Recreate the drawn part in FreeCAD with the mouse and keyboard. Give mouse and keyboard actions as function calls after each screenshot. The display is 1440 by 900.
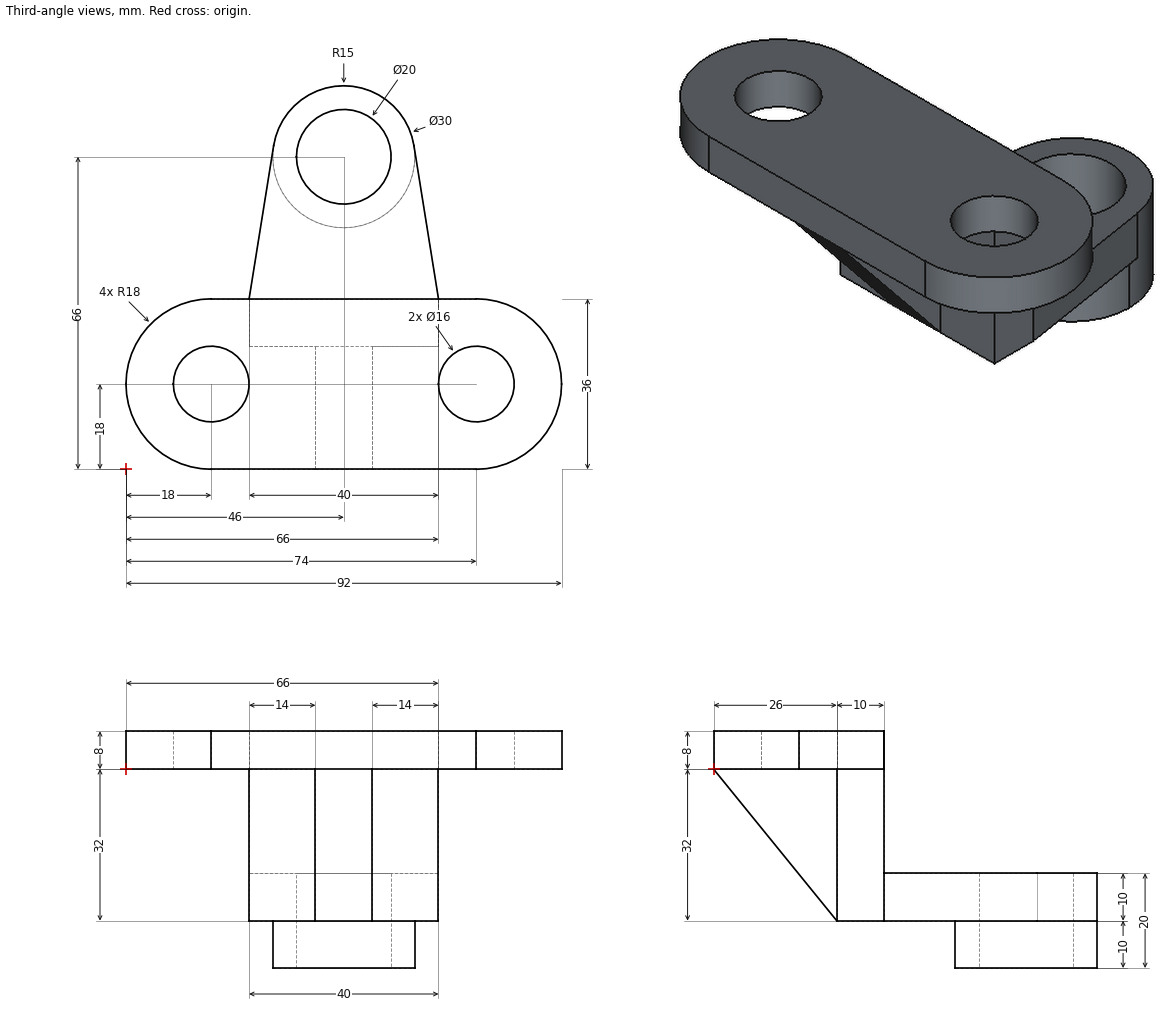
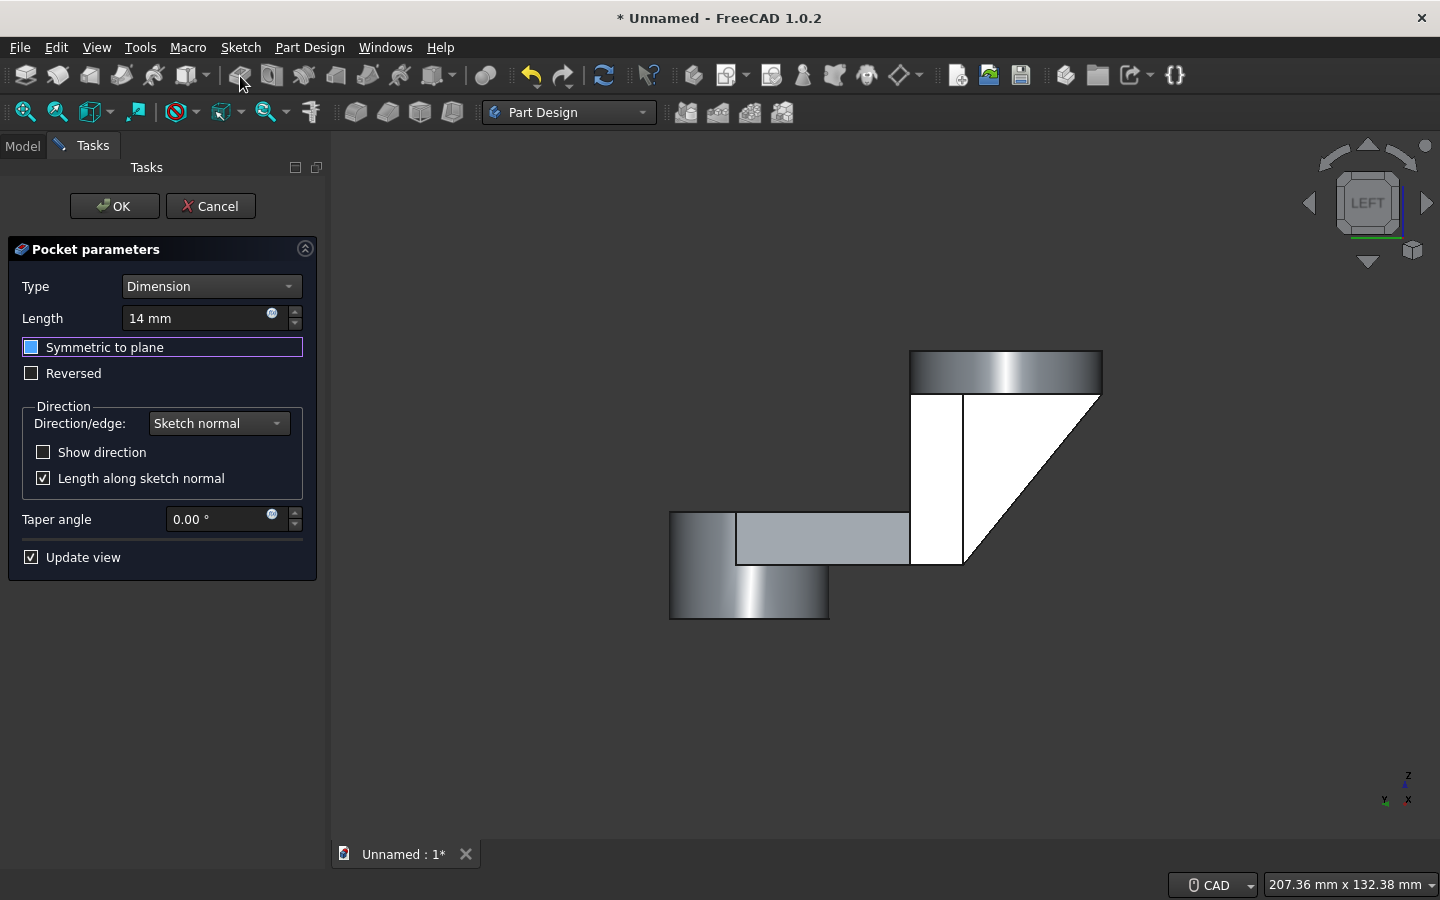
click(115, 206)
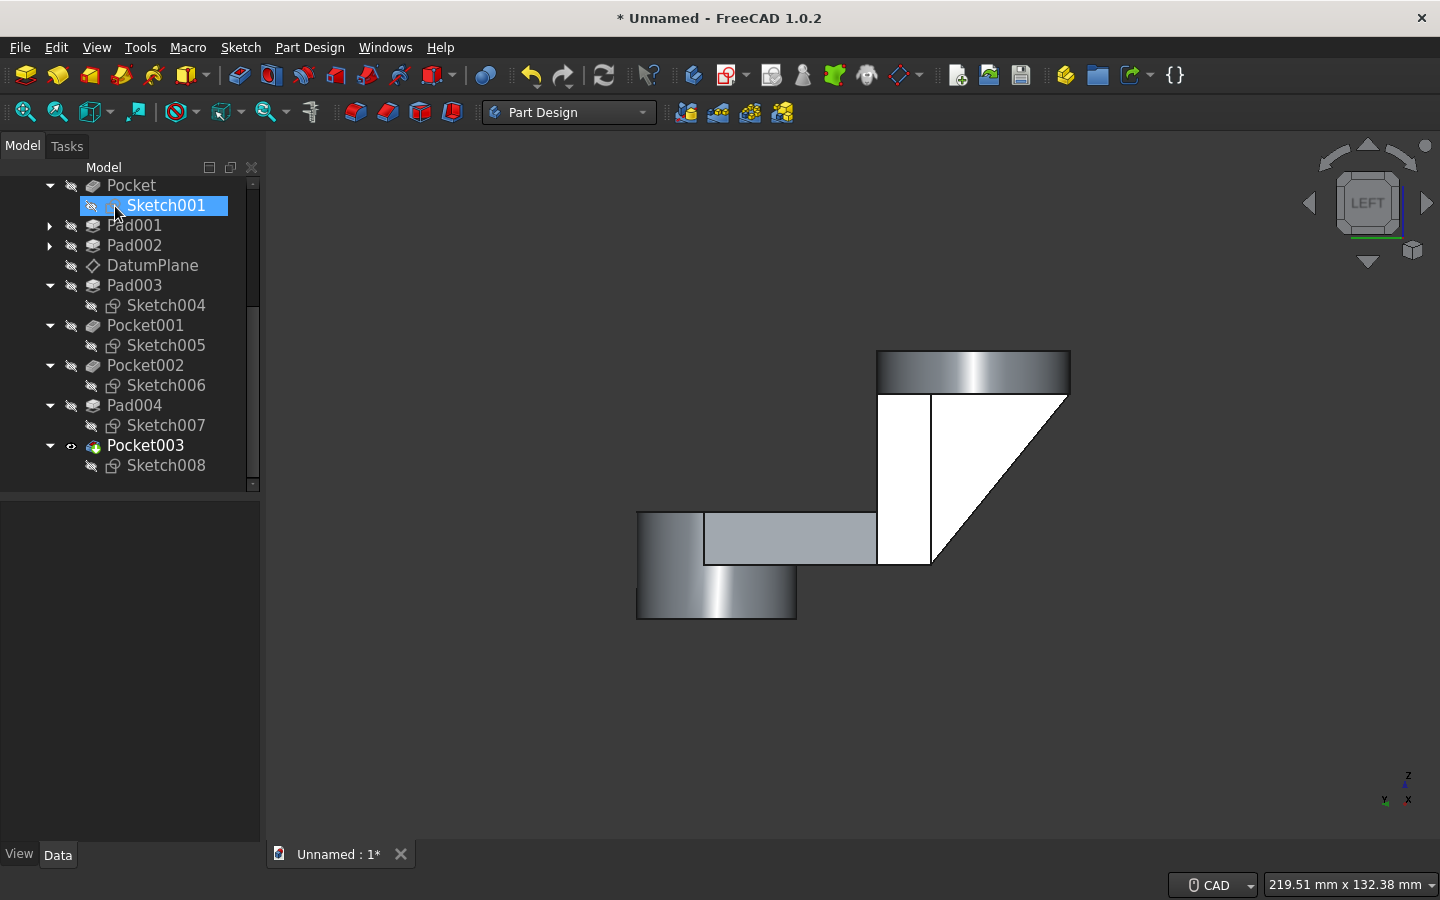
click(26, 112)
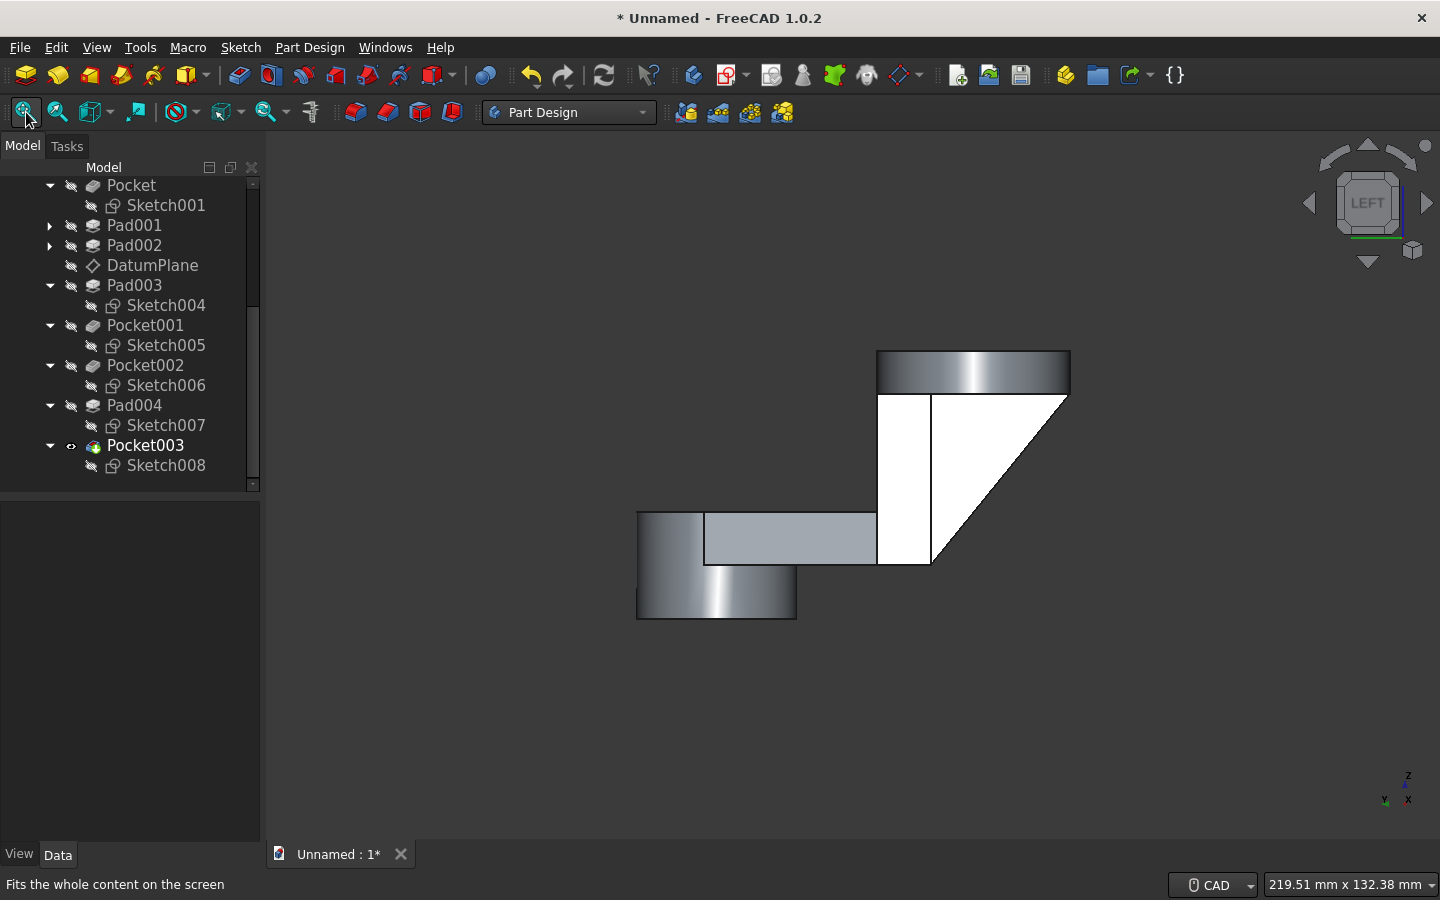
key(0)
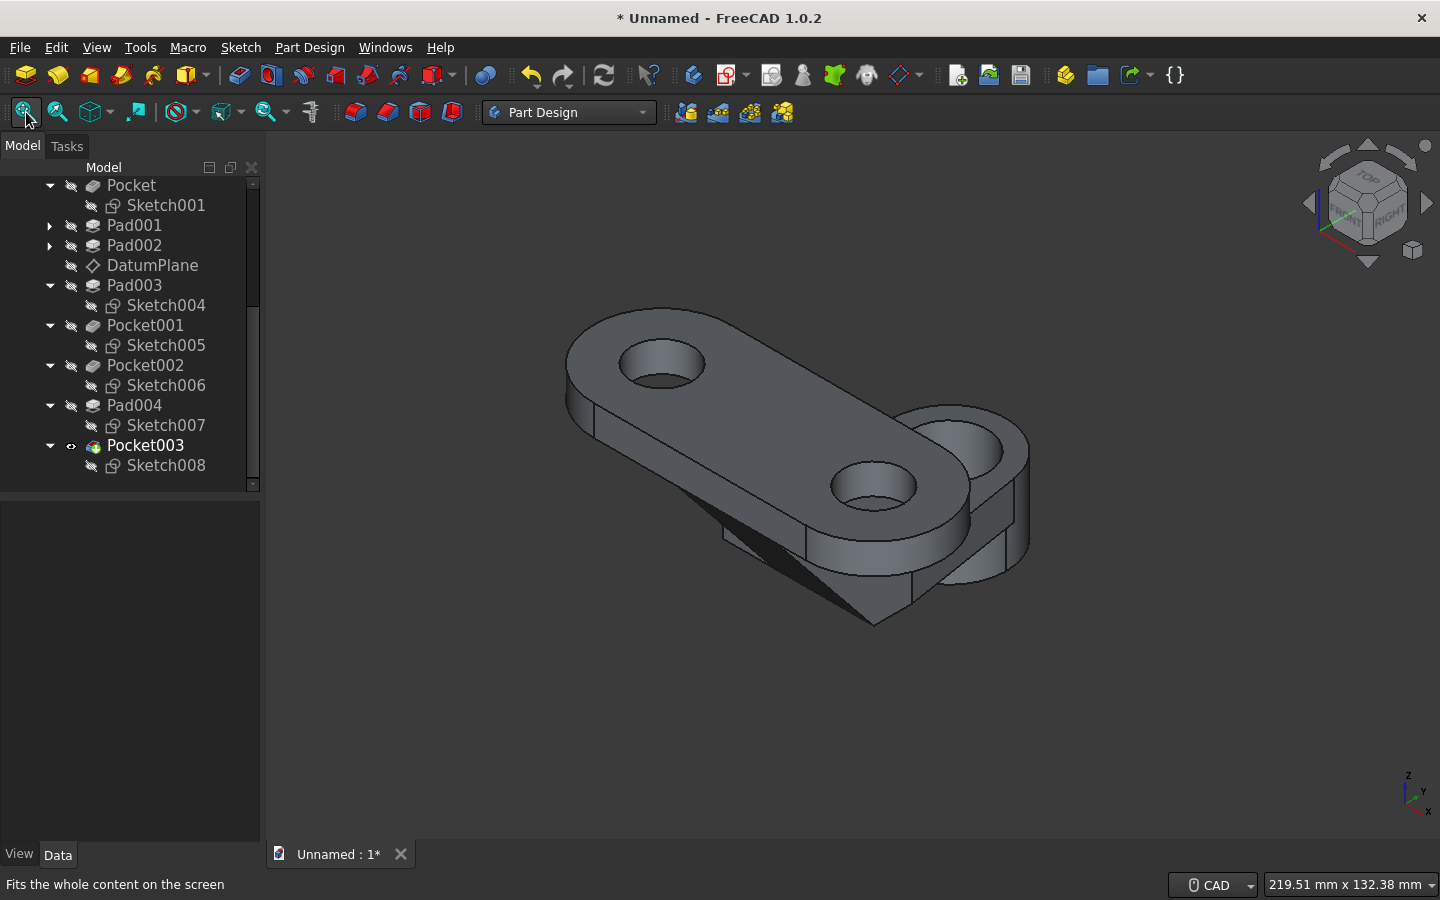
key(3)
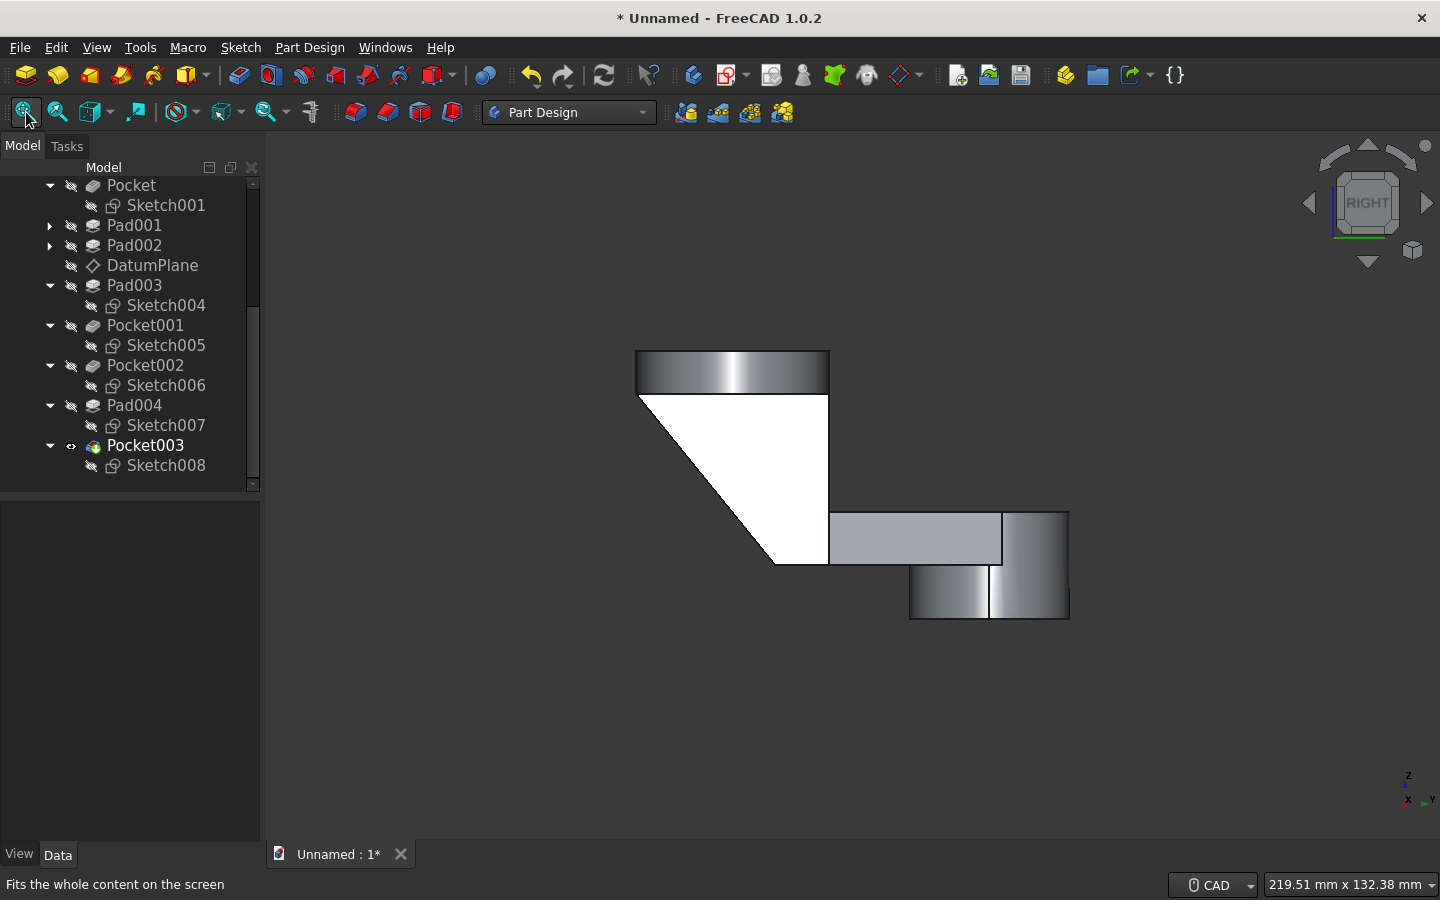
click(26, 112)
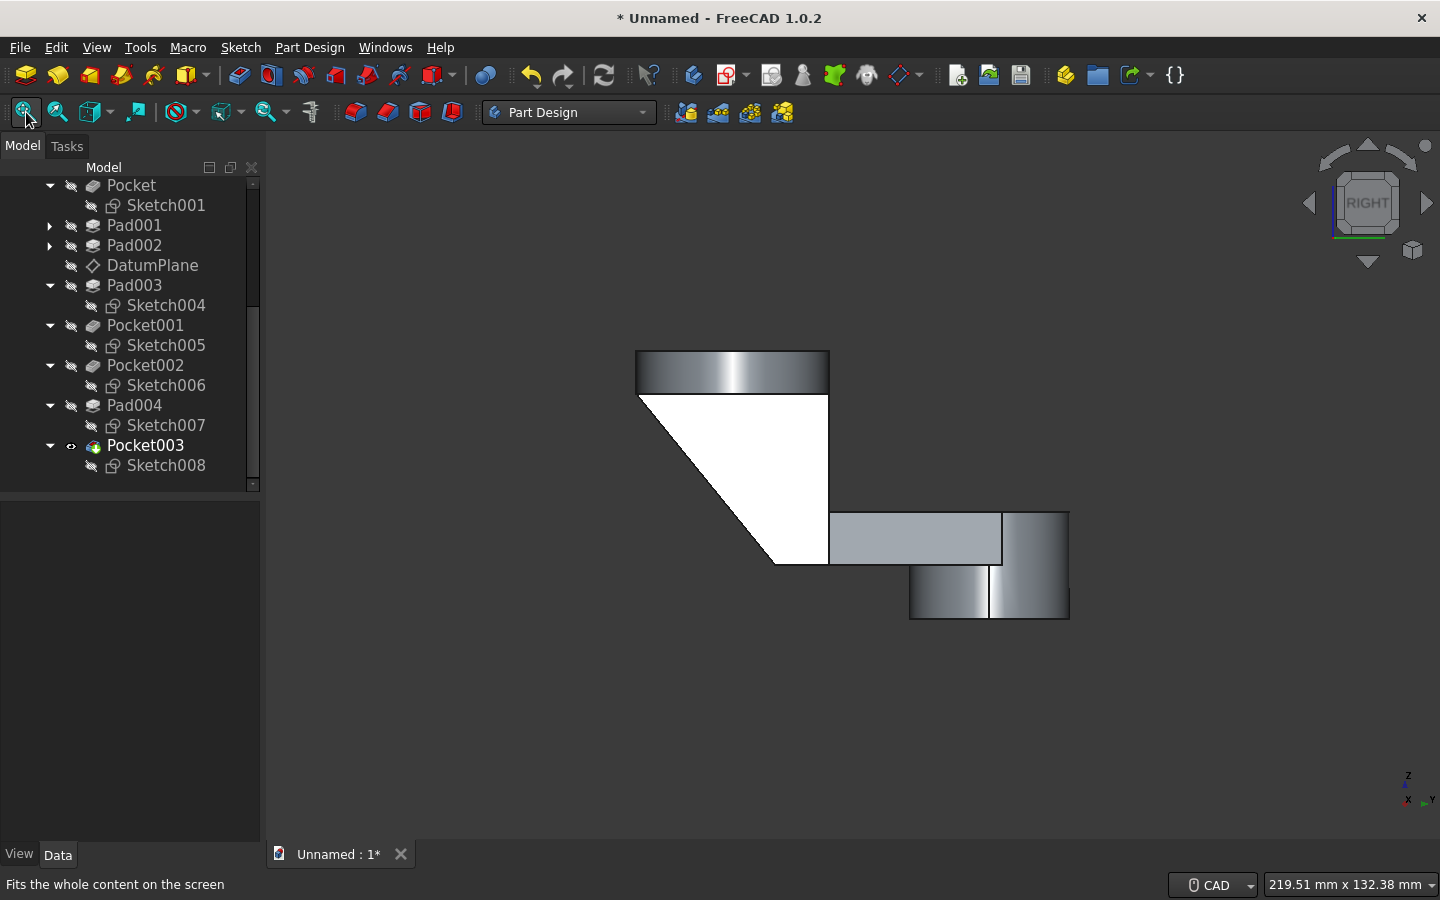
click(760, 454)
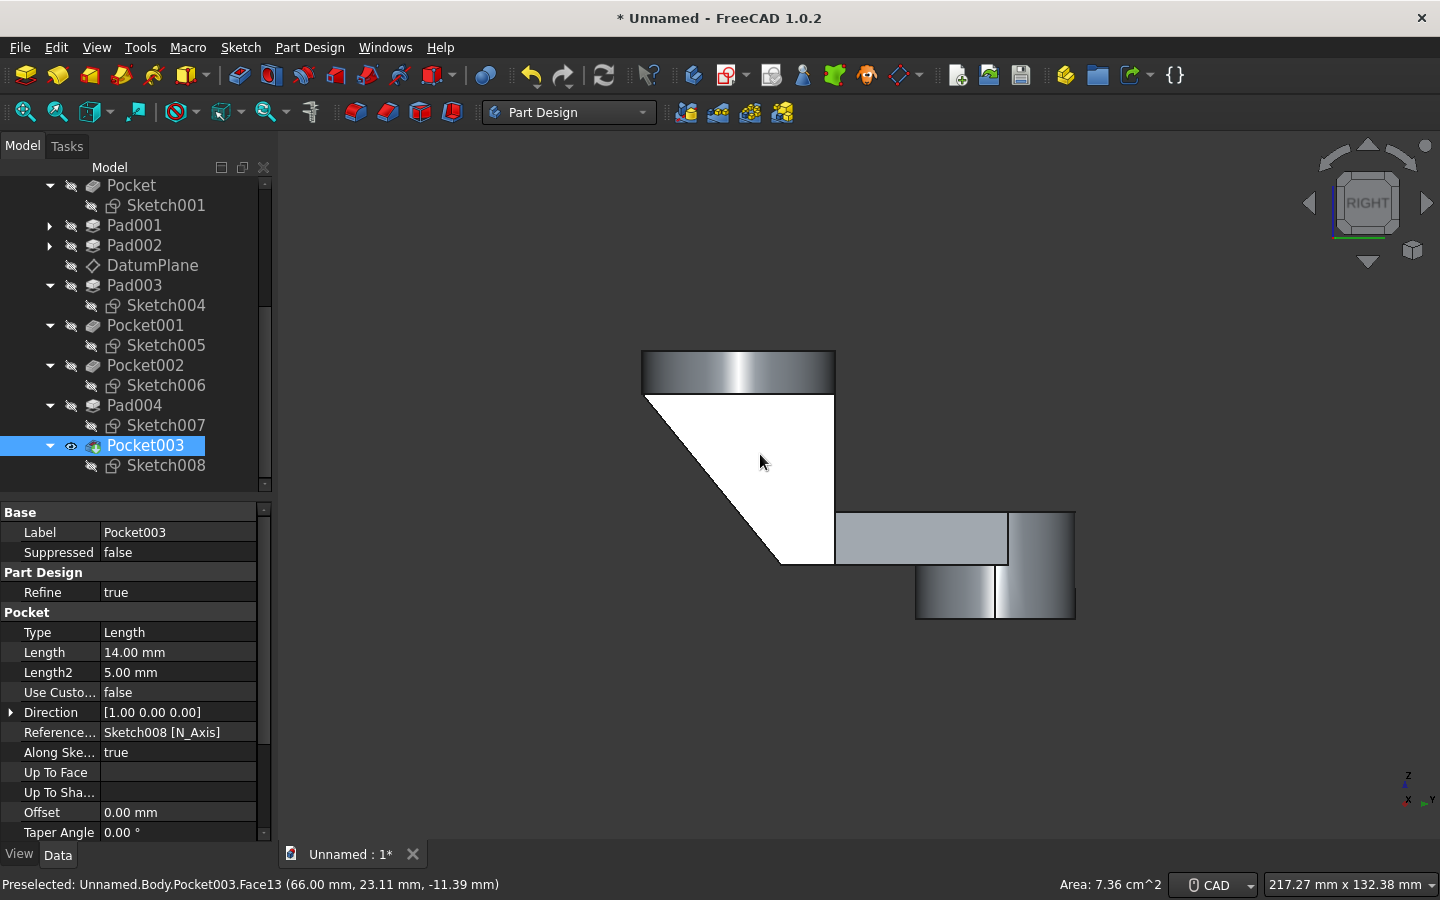
click(726, 76)